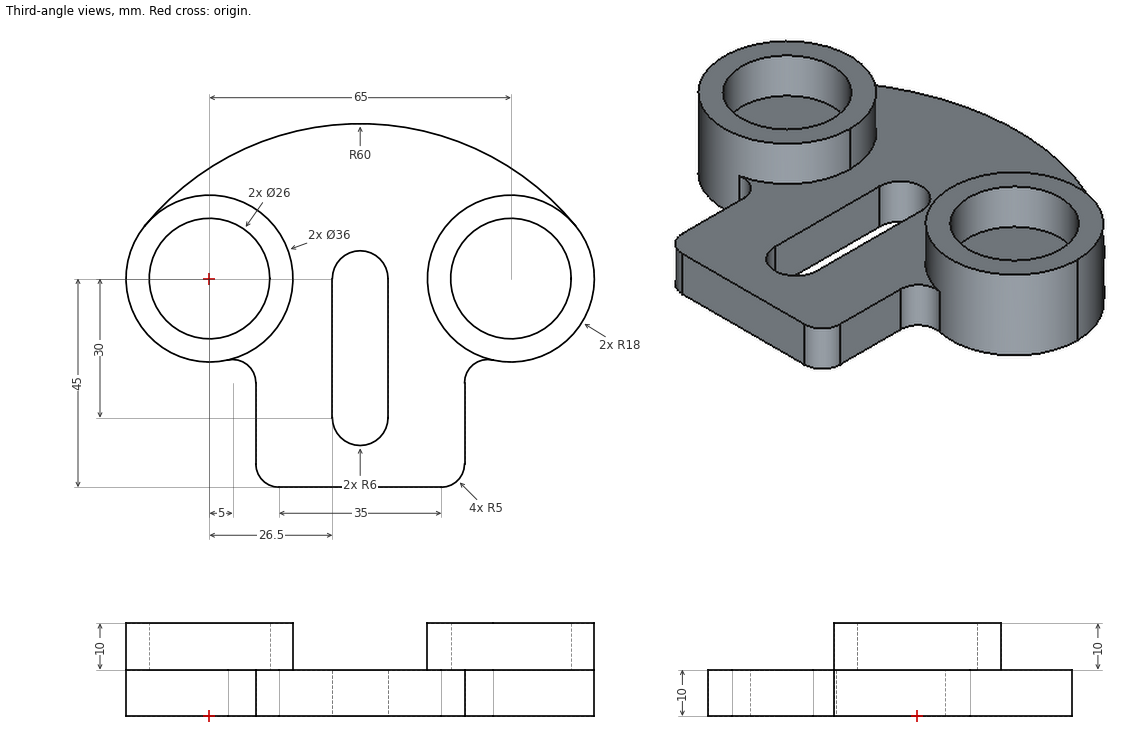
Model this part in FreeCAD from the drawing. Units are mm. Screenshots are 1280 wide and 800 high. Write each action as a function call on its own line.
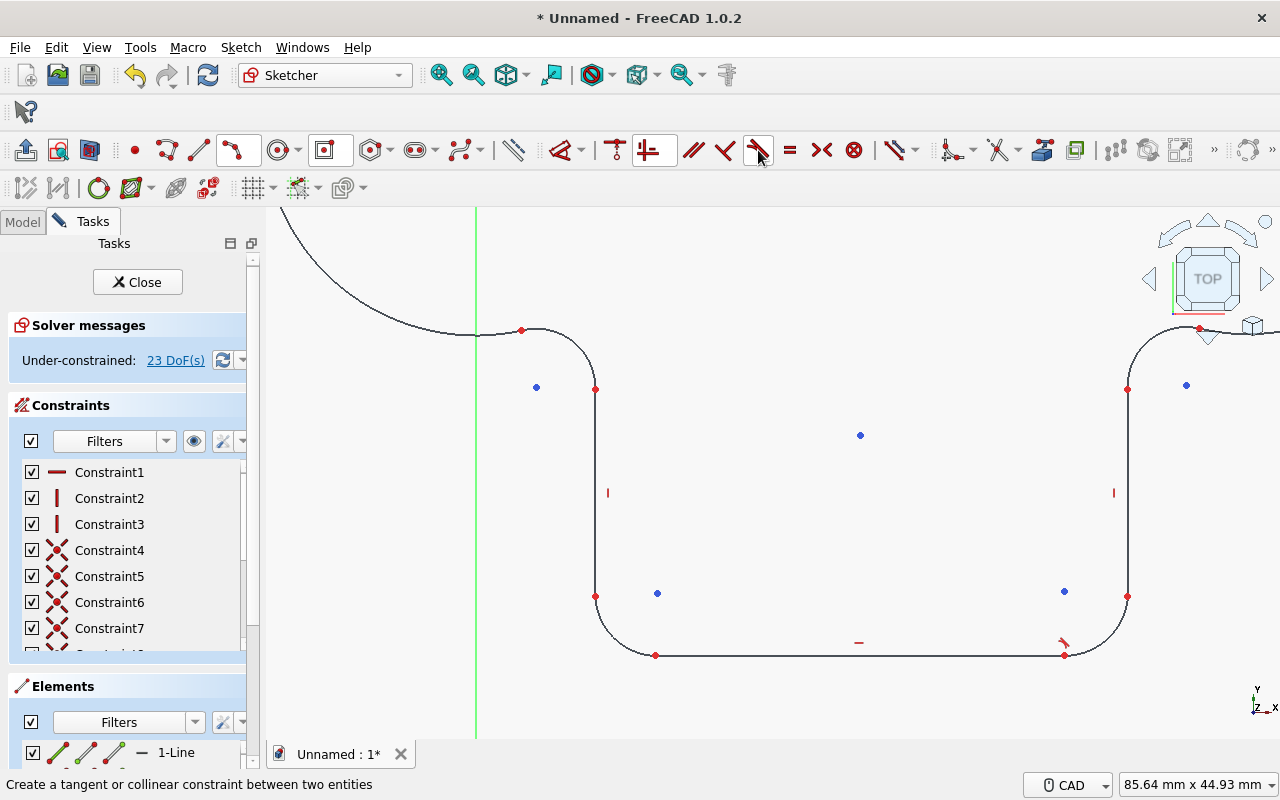
click(778, 656)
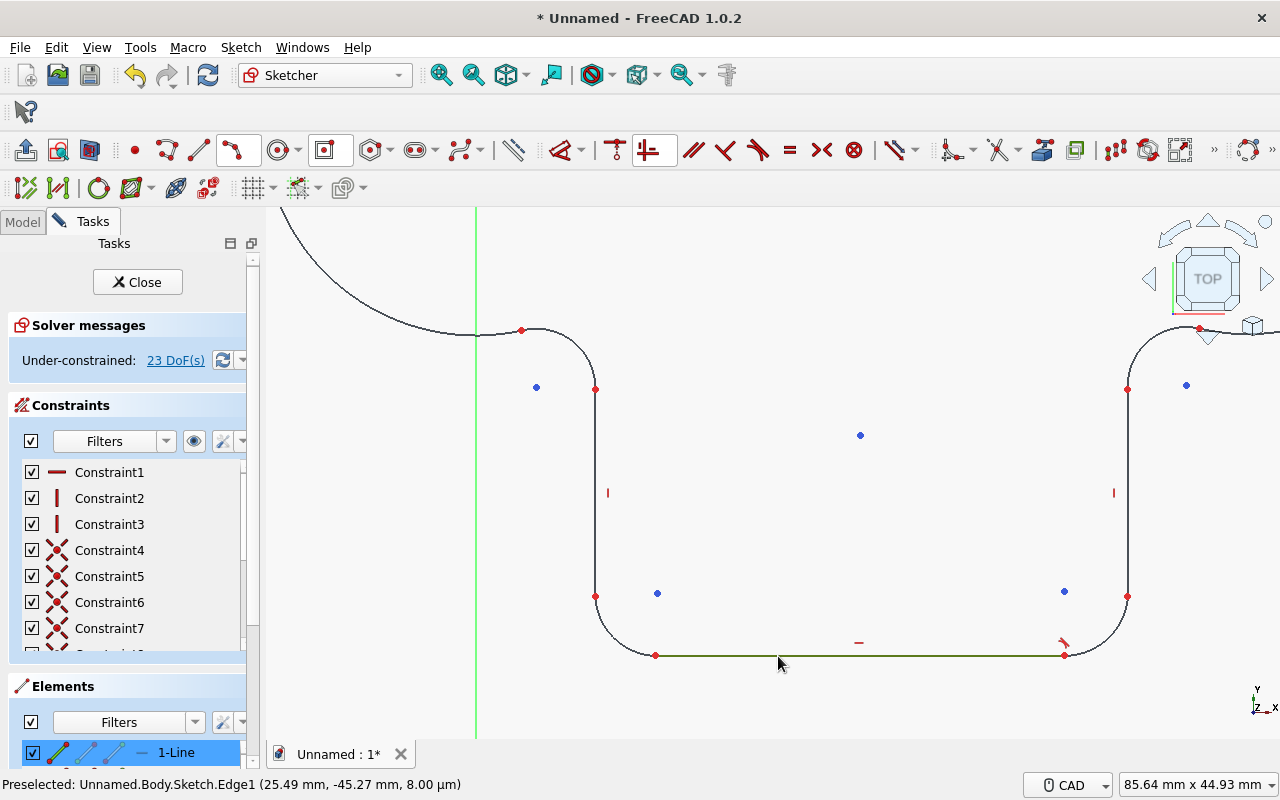
click(603, 623)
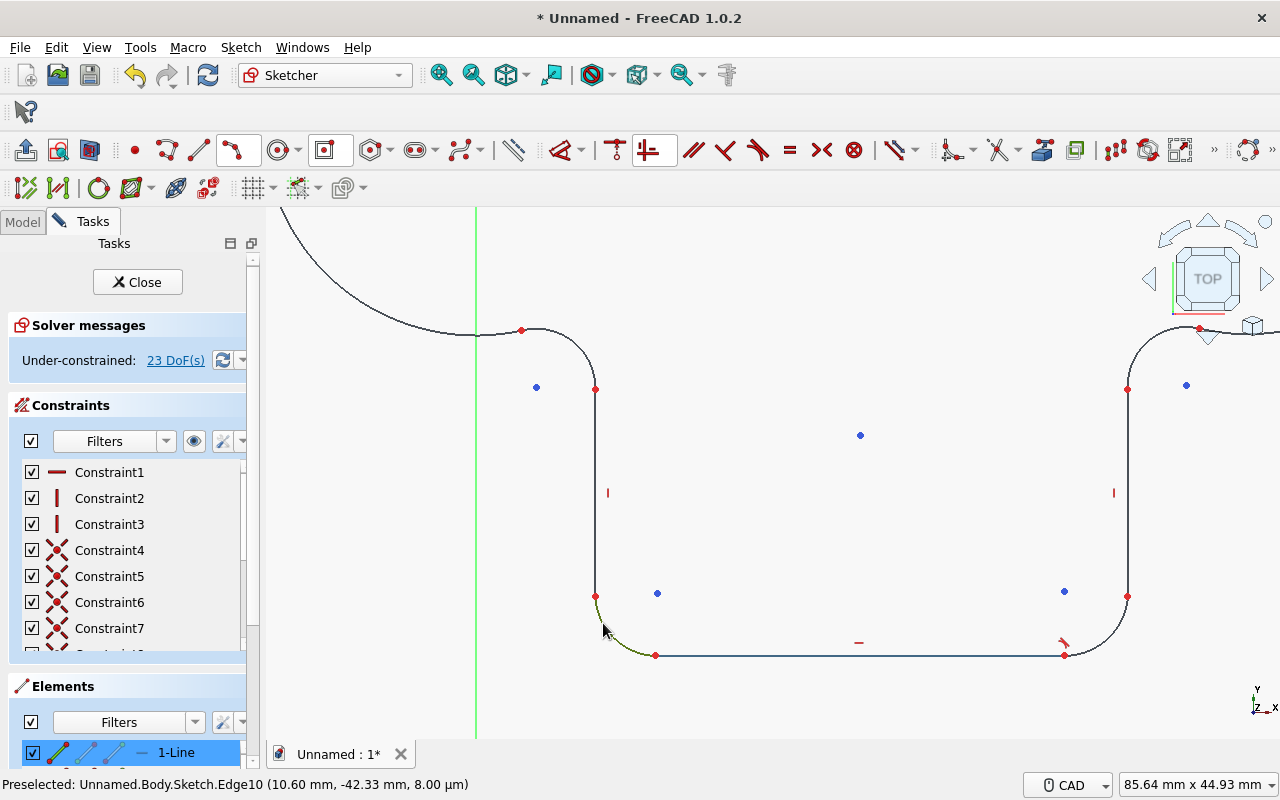
click(758, 150)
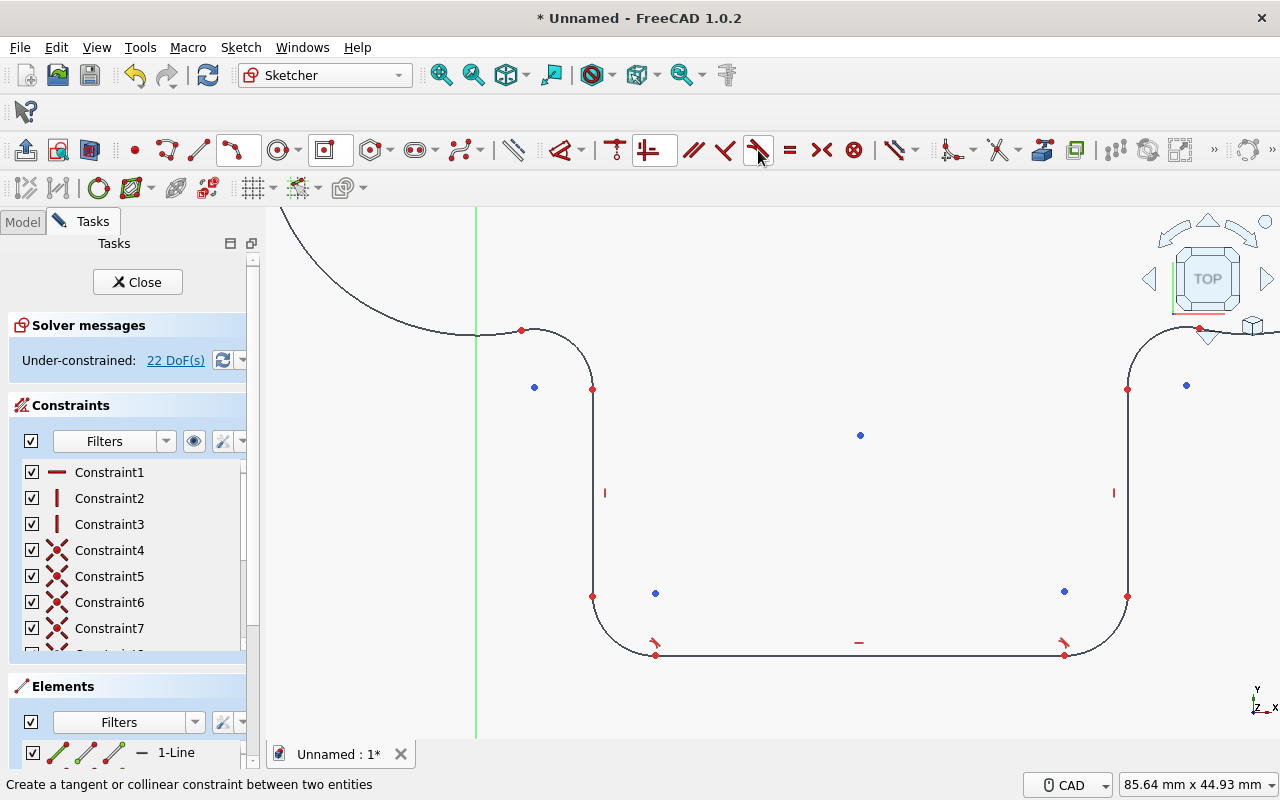
scroll(613, 638, down, 5)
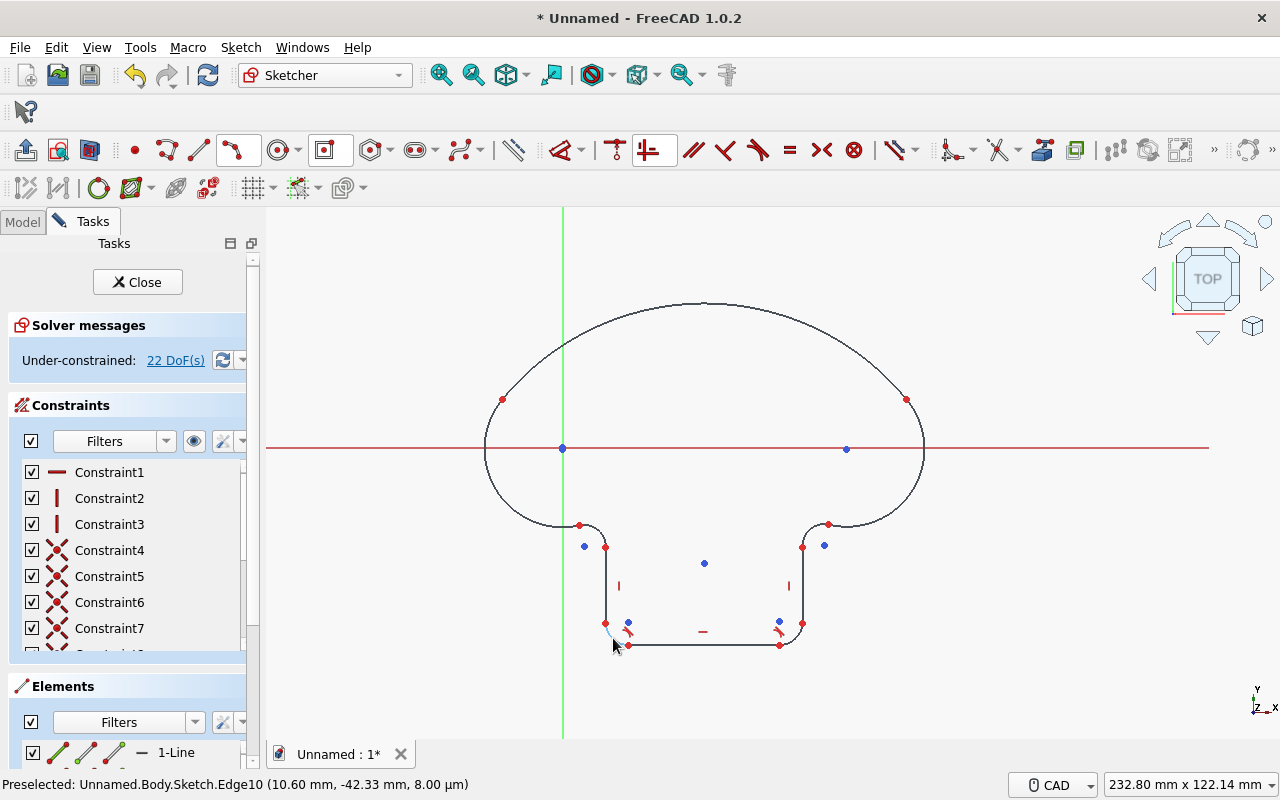
click(803, 600)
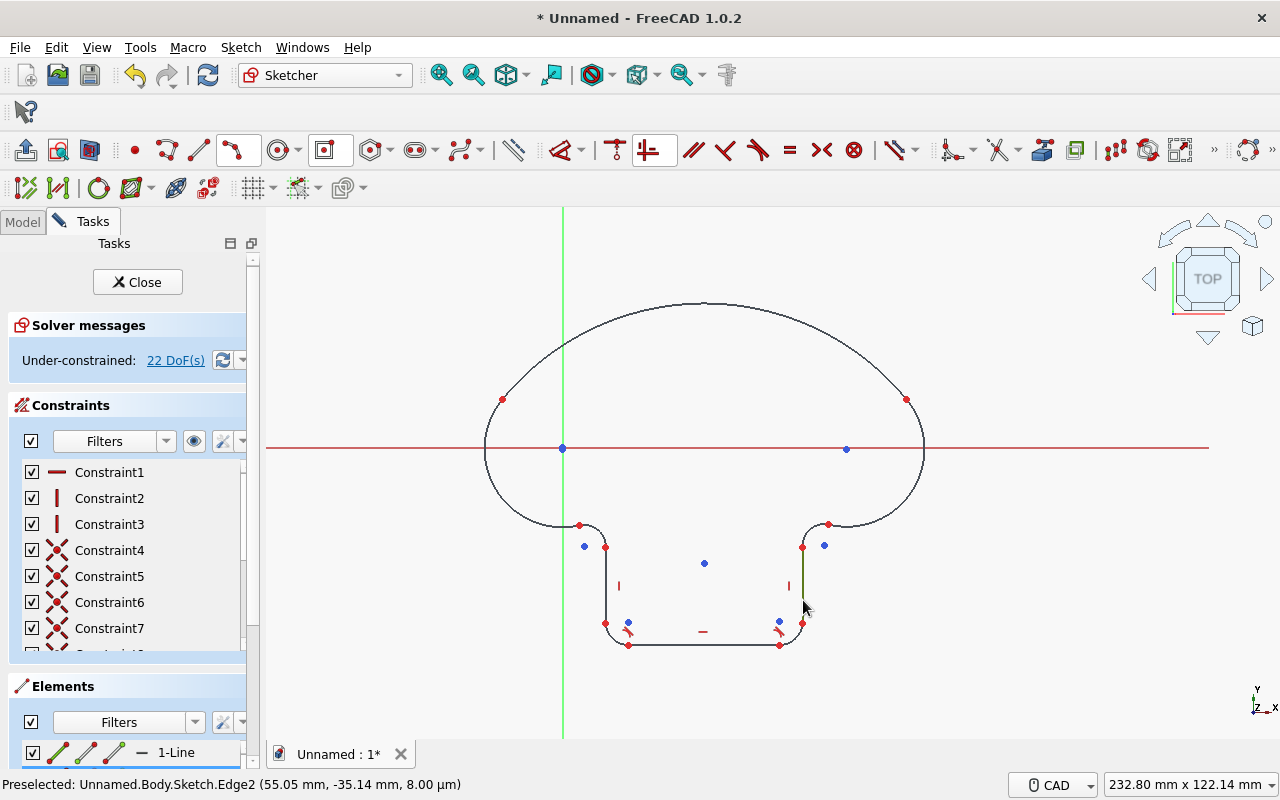
scroll(789, 643, up, 2)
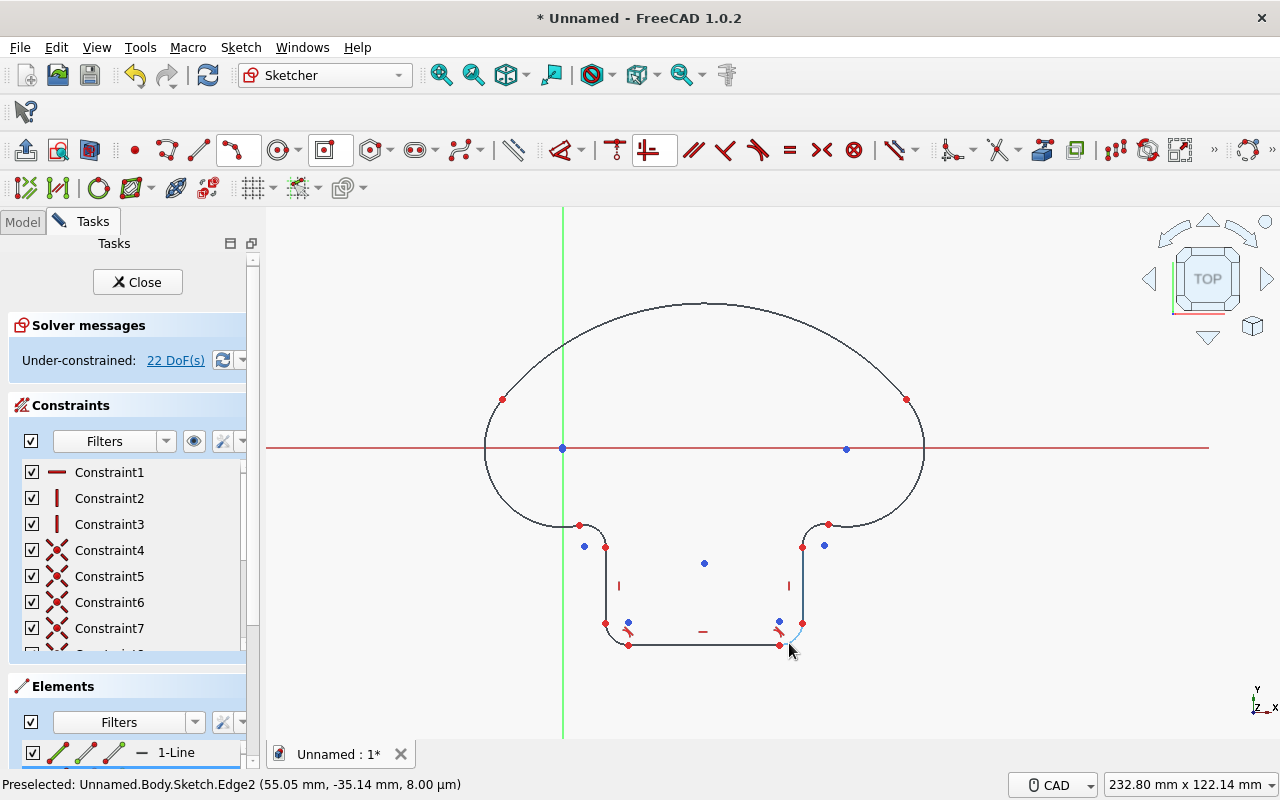
click(789, 642)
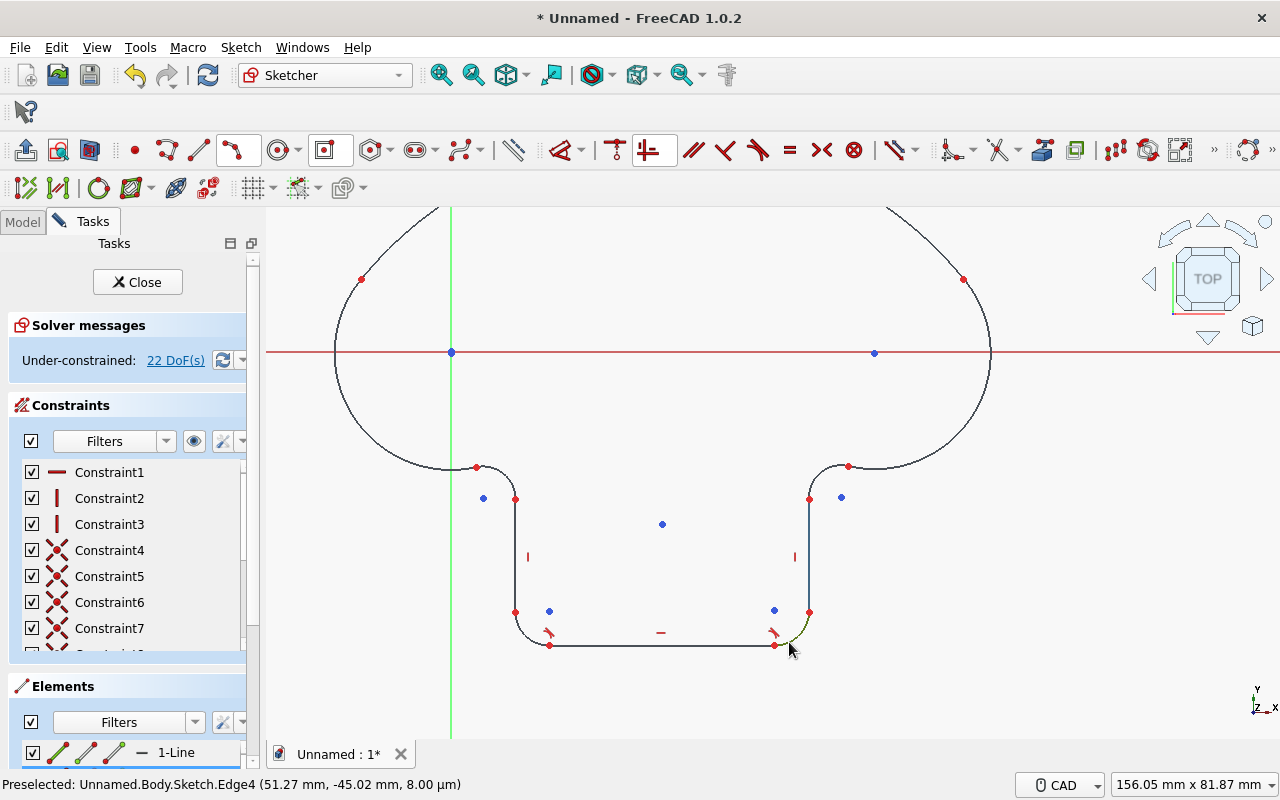
click(758, 150)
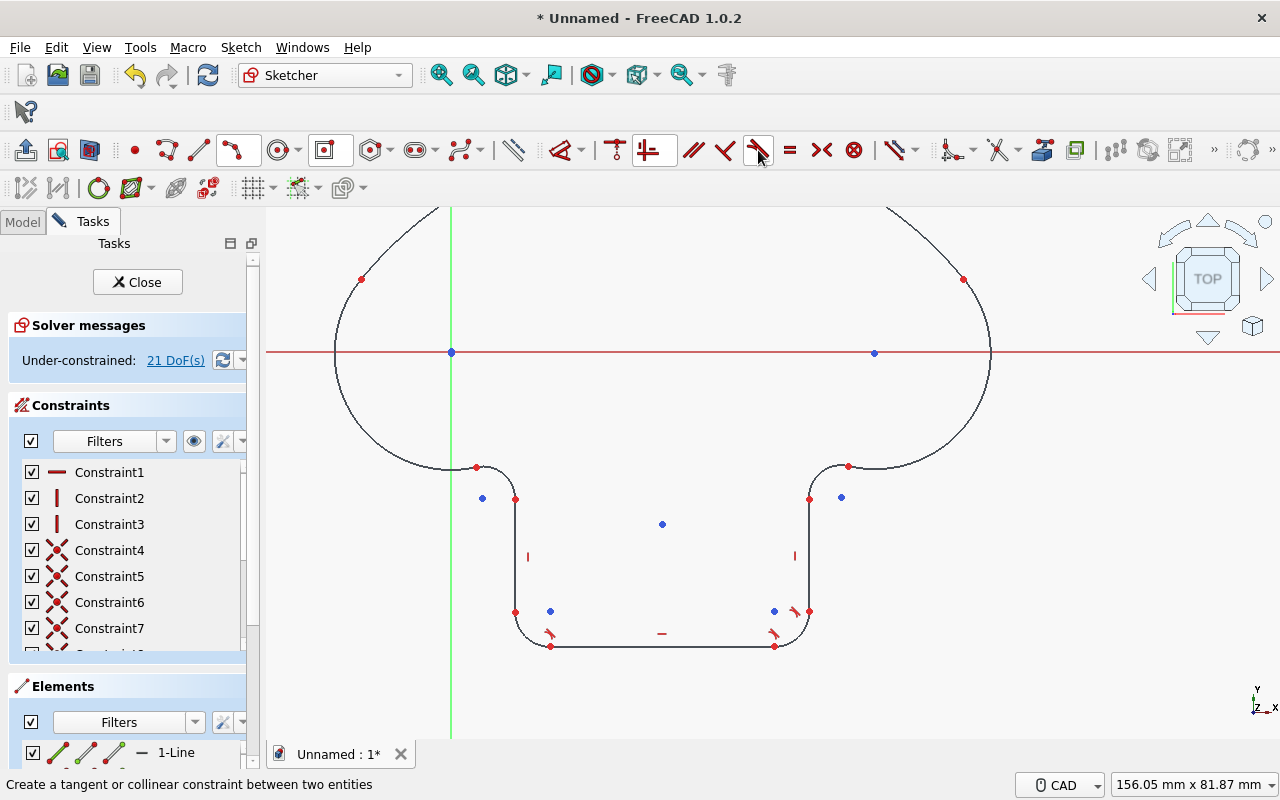
click(809, 578)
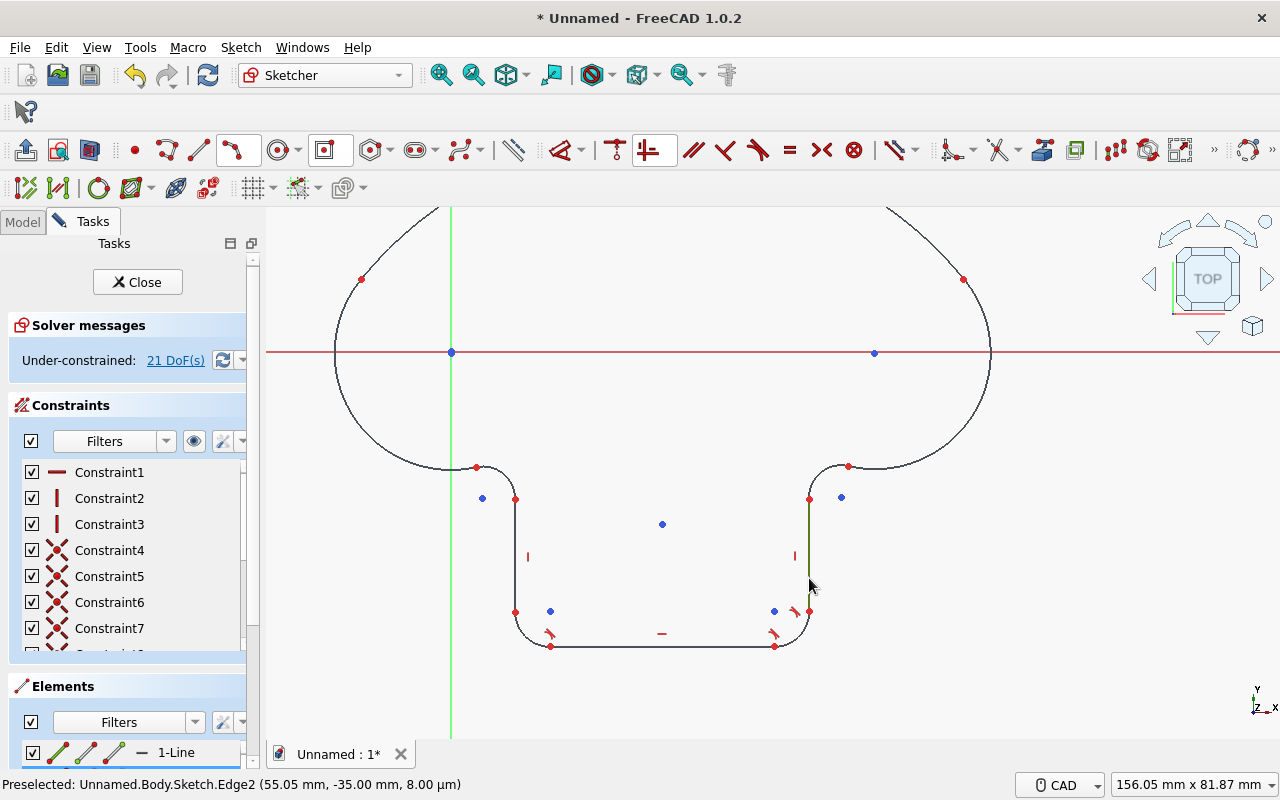
click(831, 467)